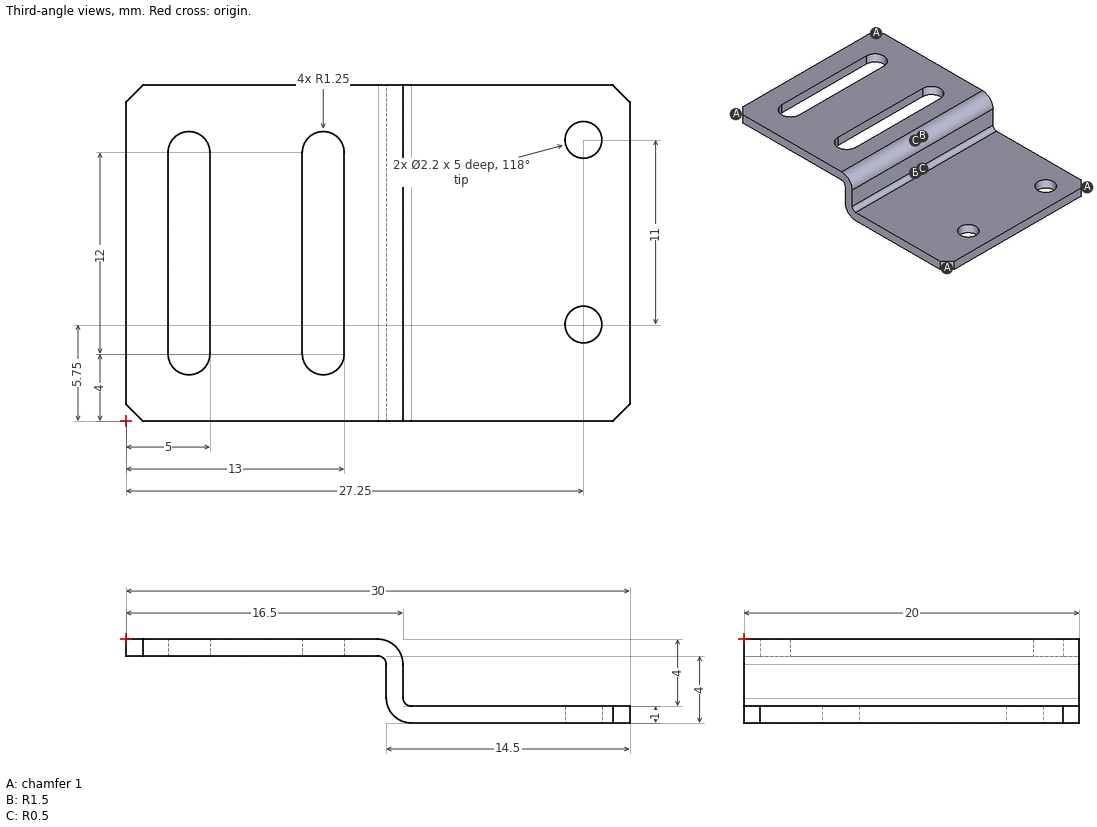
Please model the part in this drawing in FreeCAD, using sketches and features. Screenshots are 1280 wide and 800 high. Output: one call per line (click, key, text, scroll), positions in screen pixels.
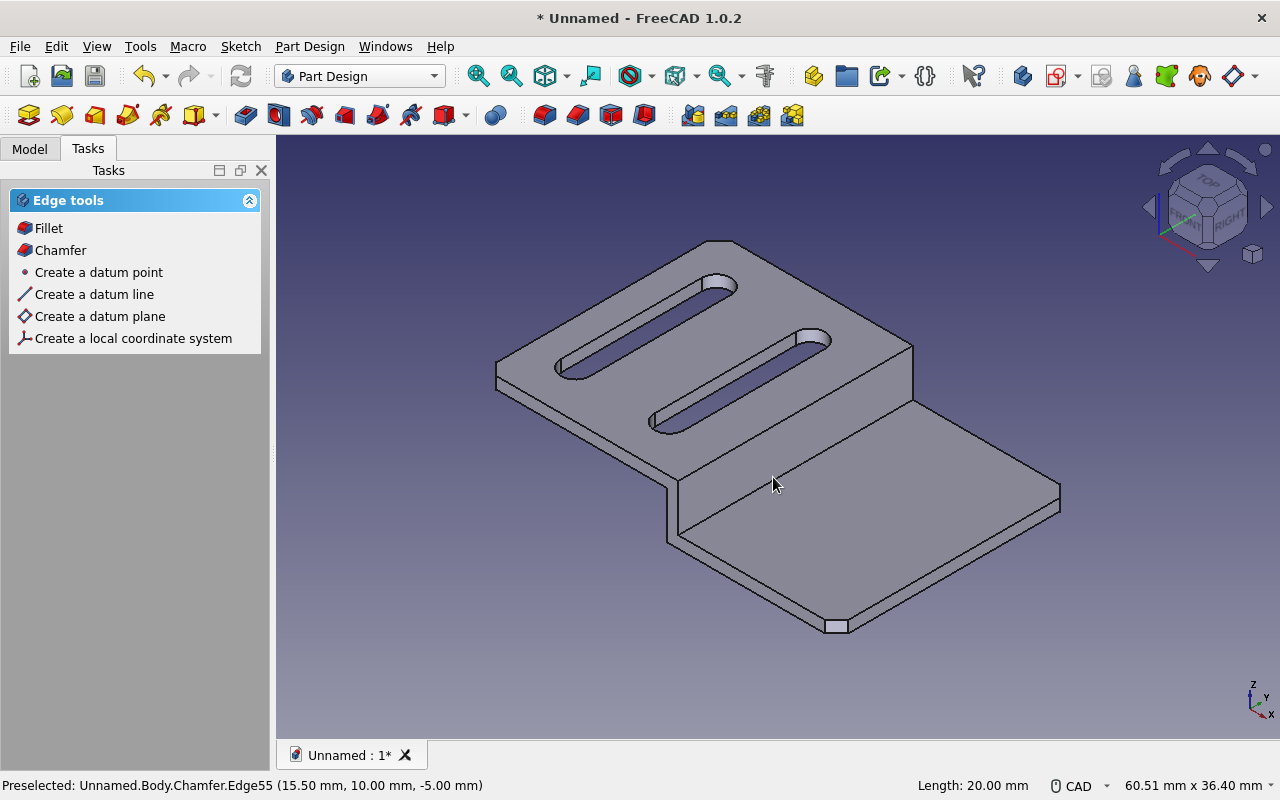
click(796, 412, ctrl)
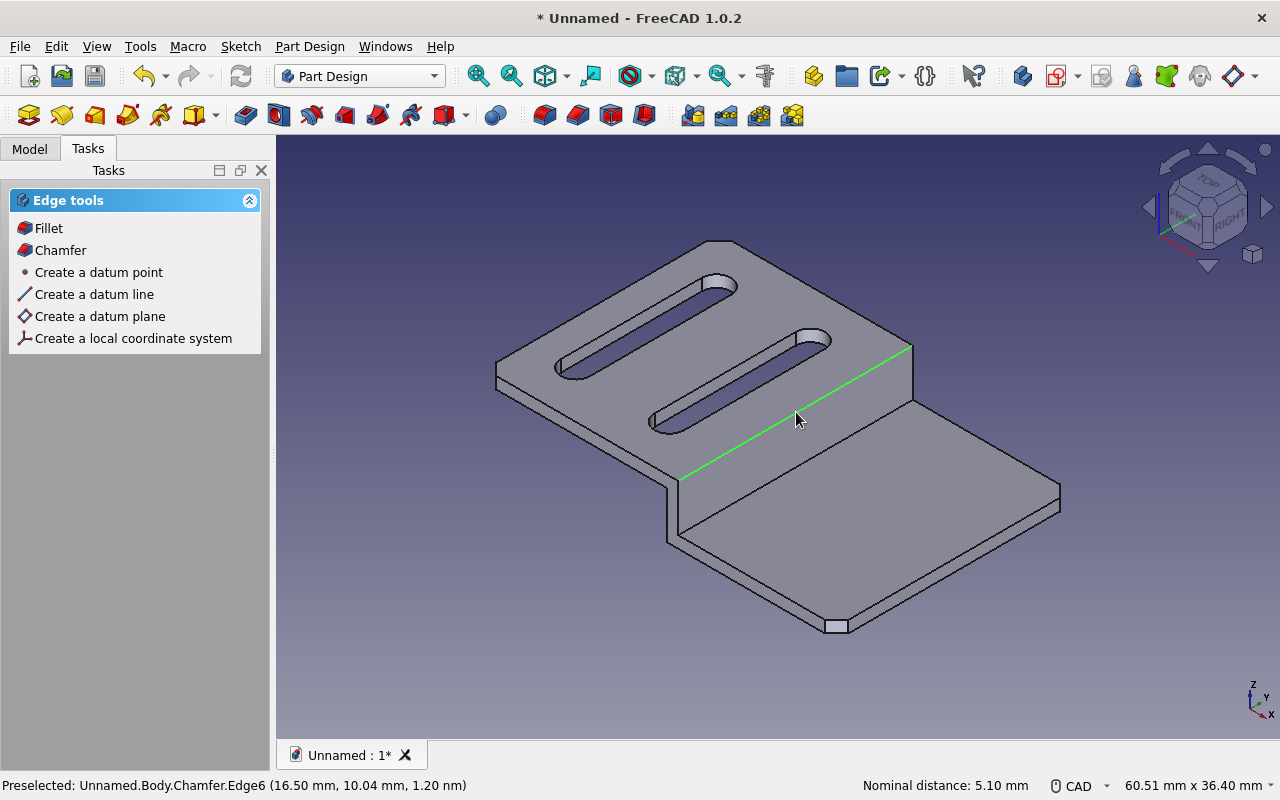
click(545, 116)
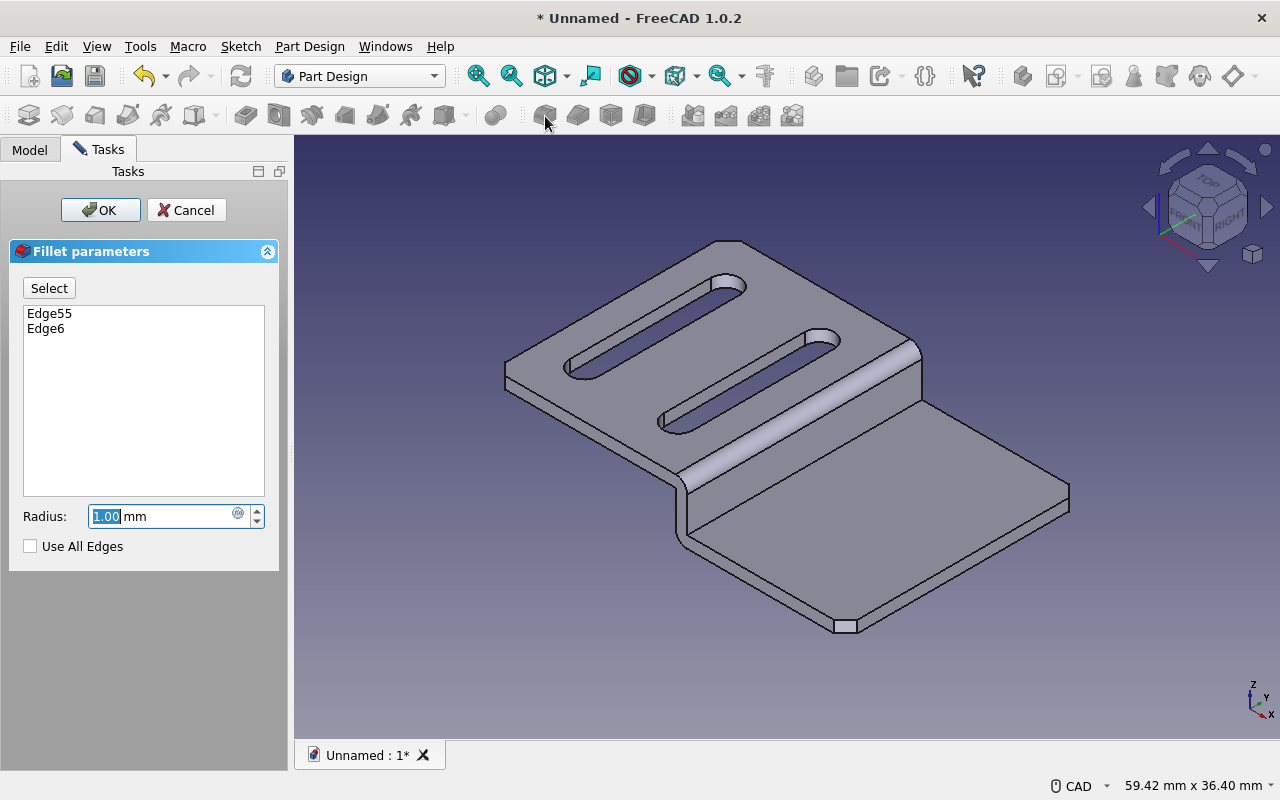
text(1.5)
key(Tab)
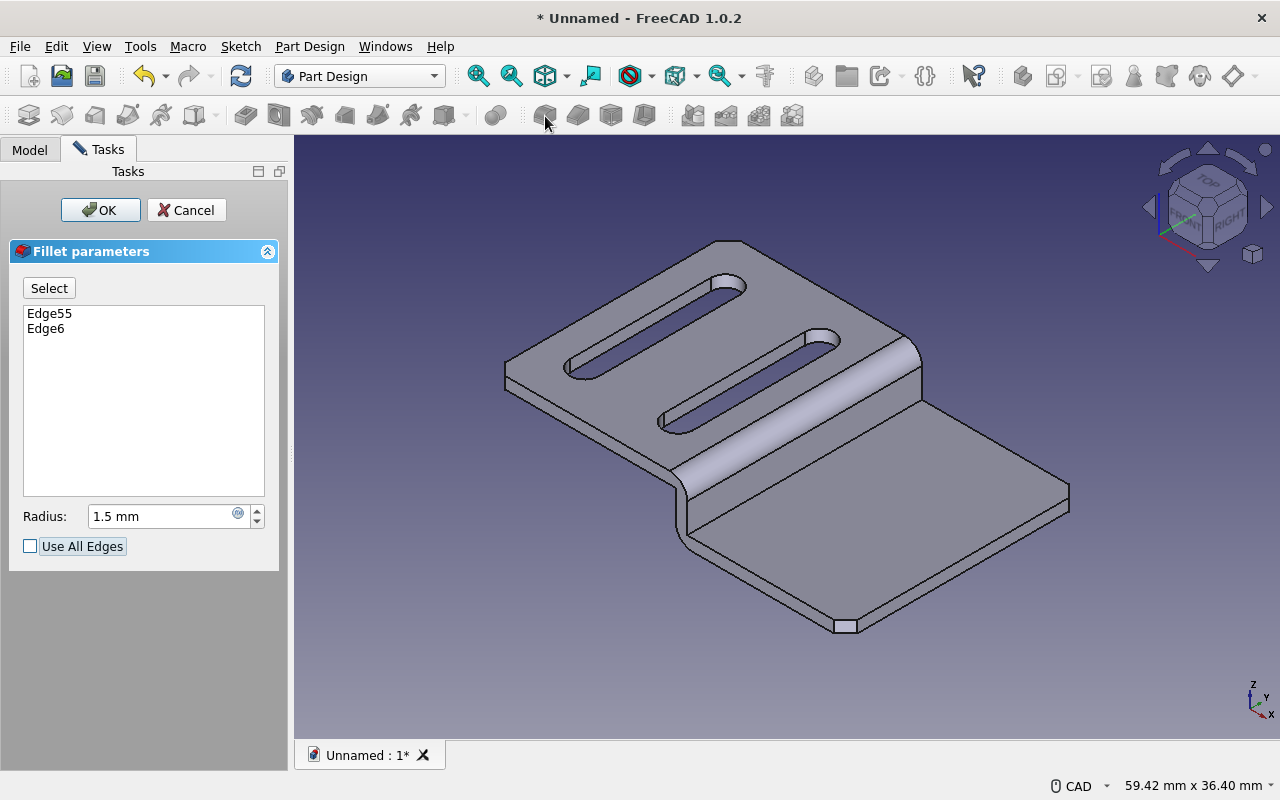
click(101, 210)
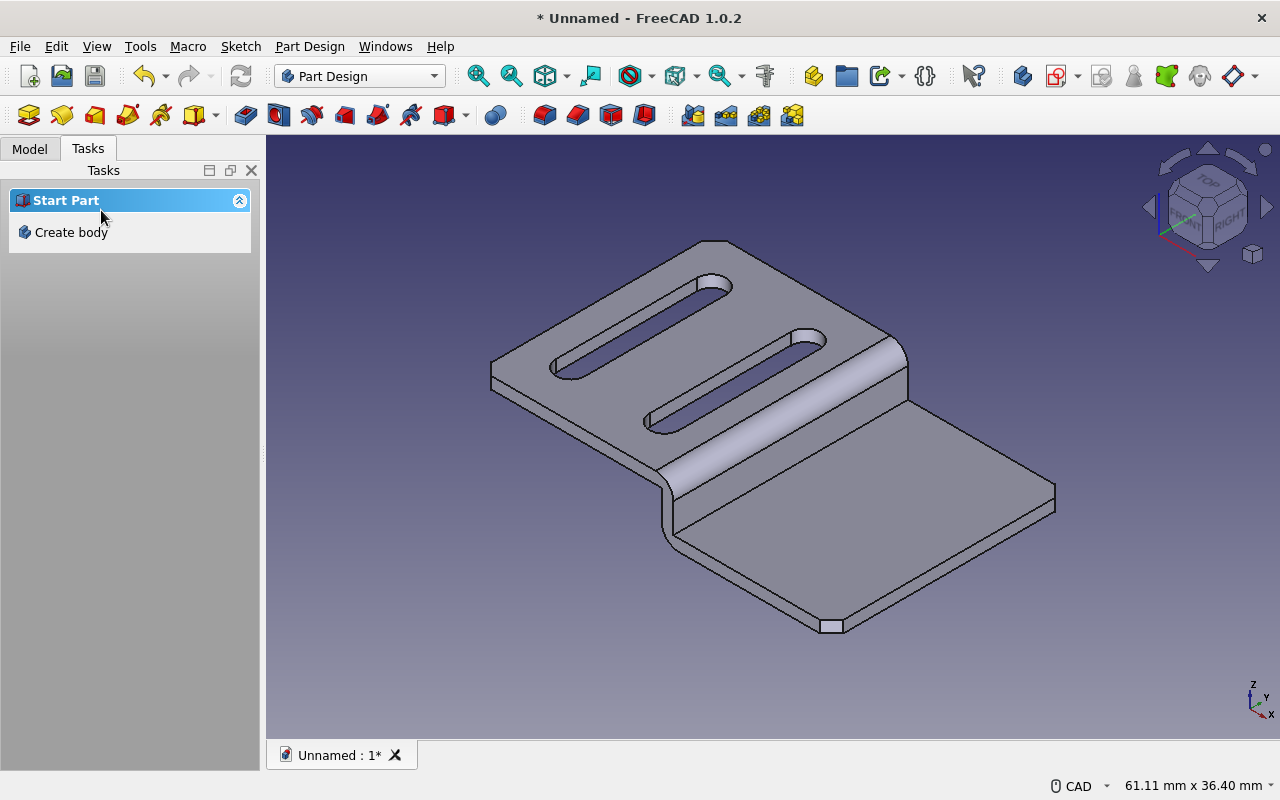
key(2)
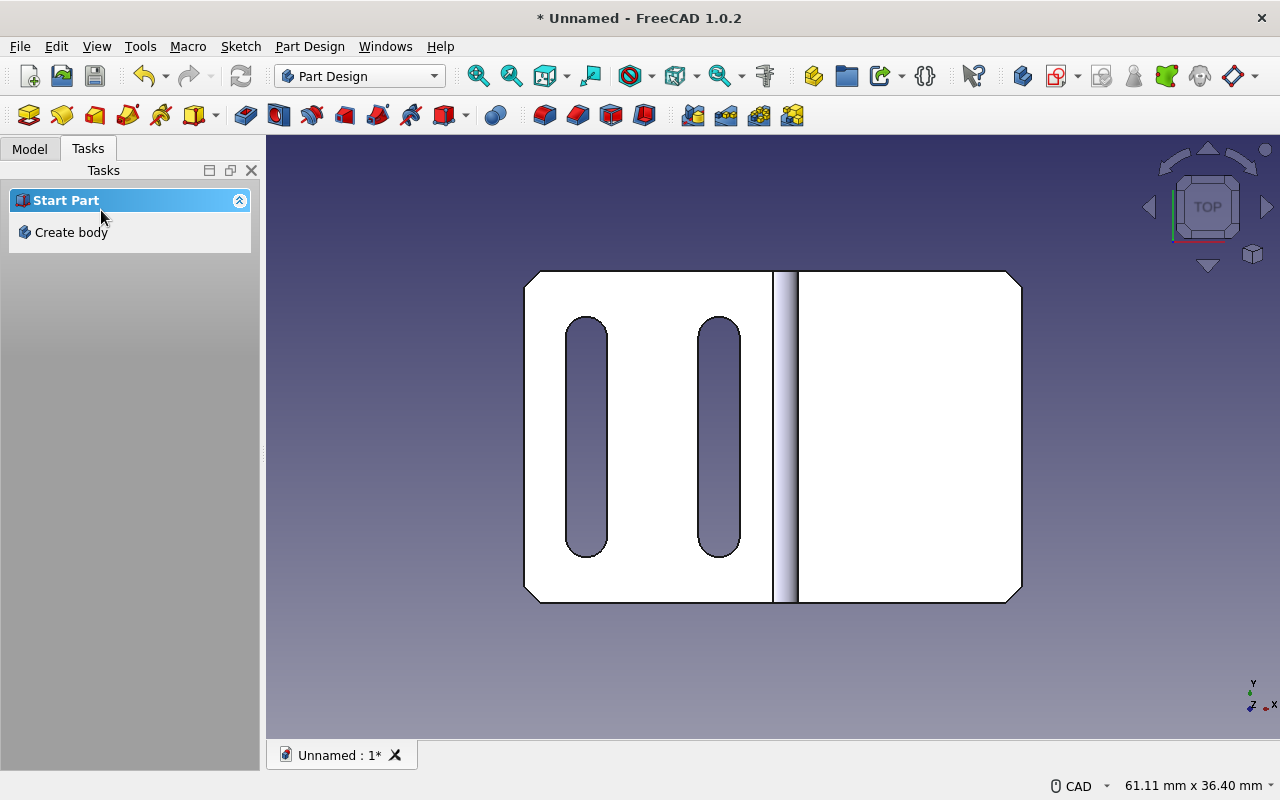
key(0)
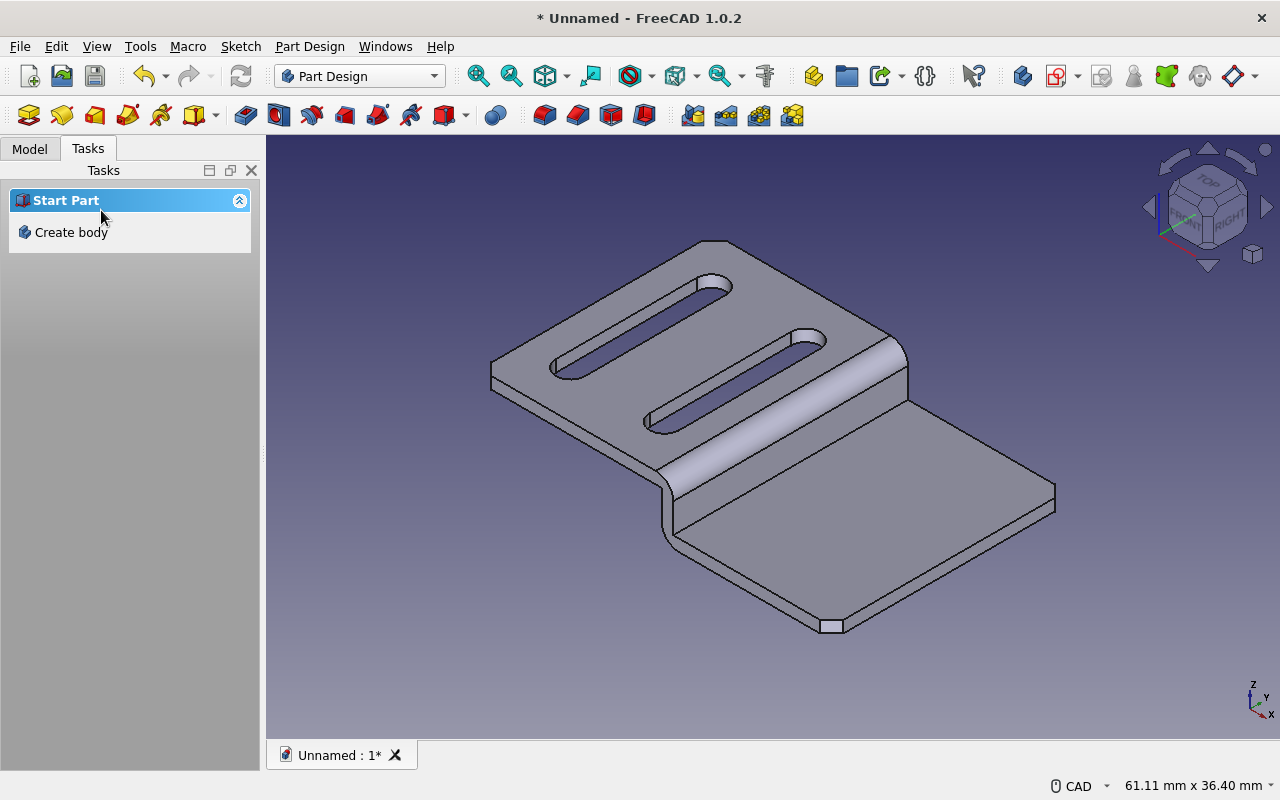
key(1)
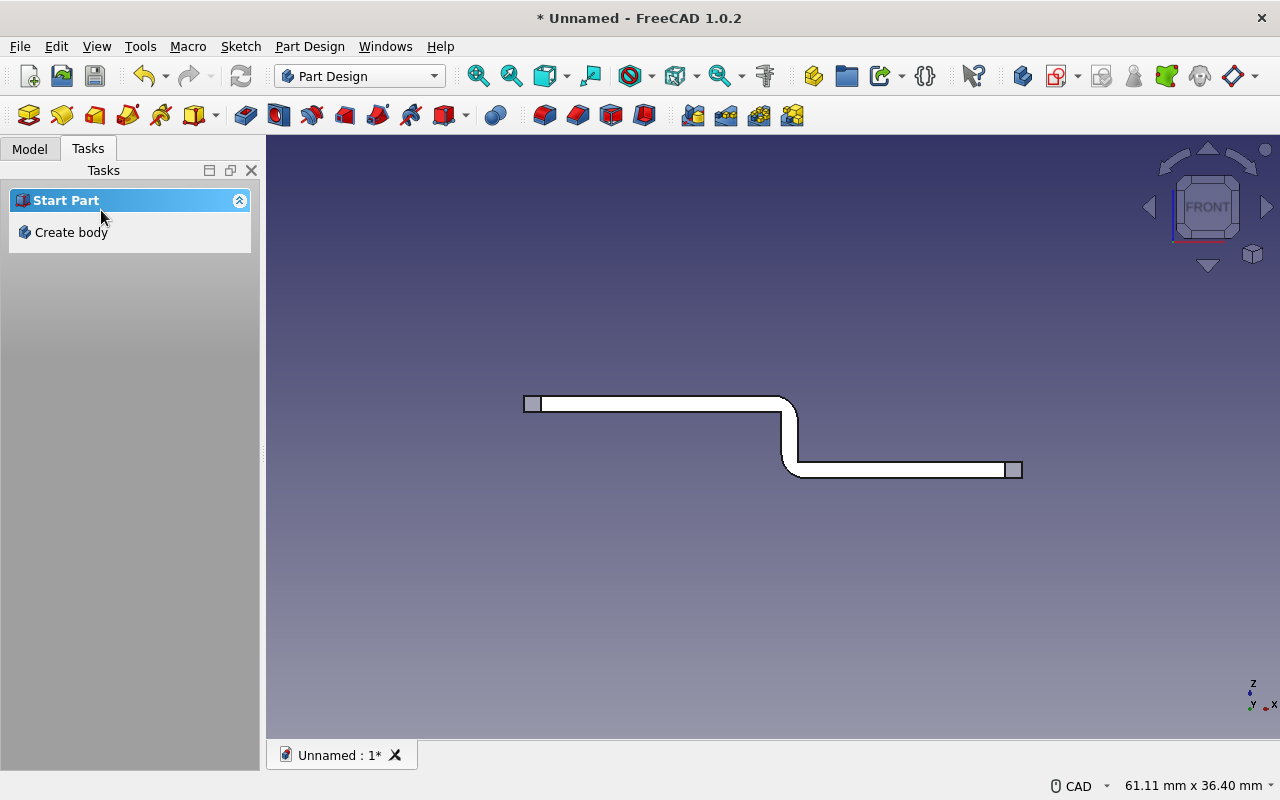
key(3)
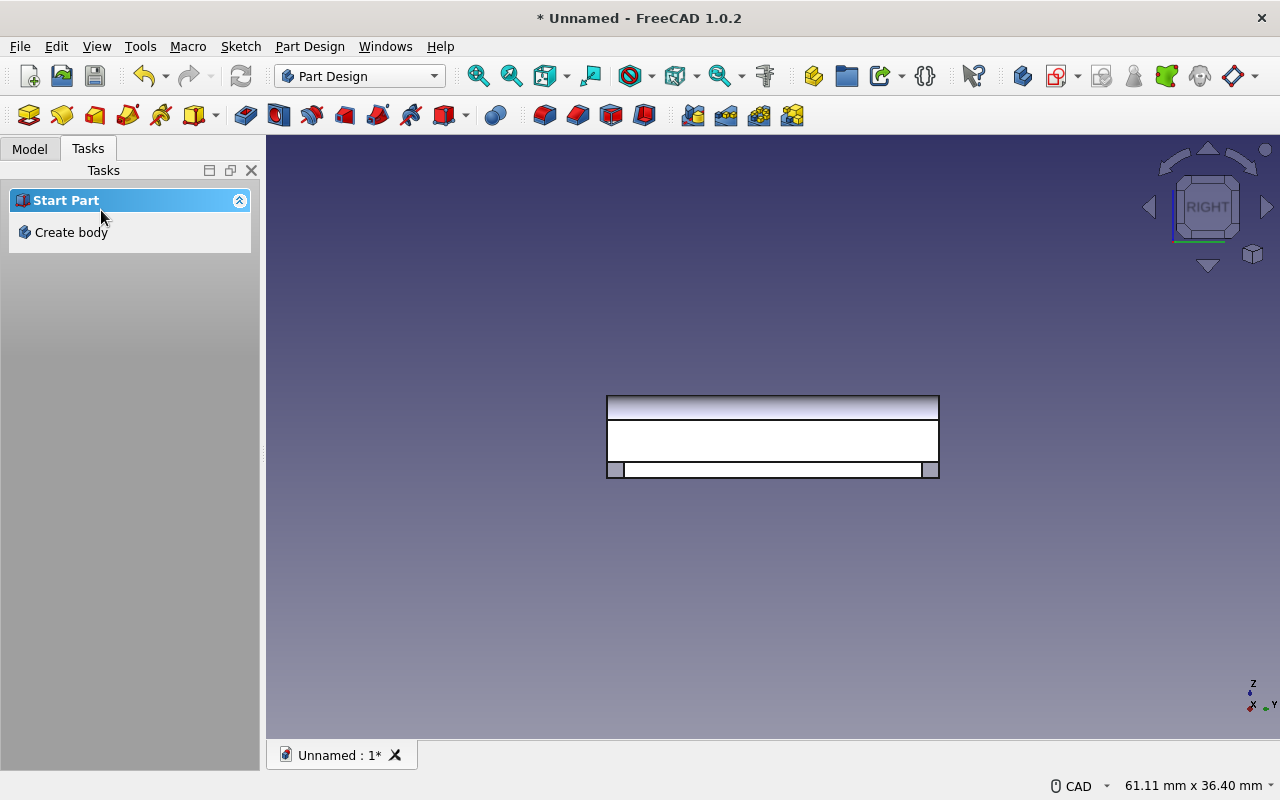
click(479, 76)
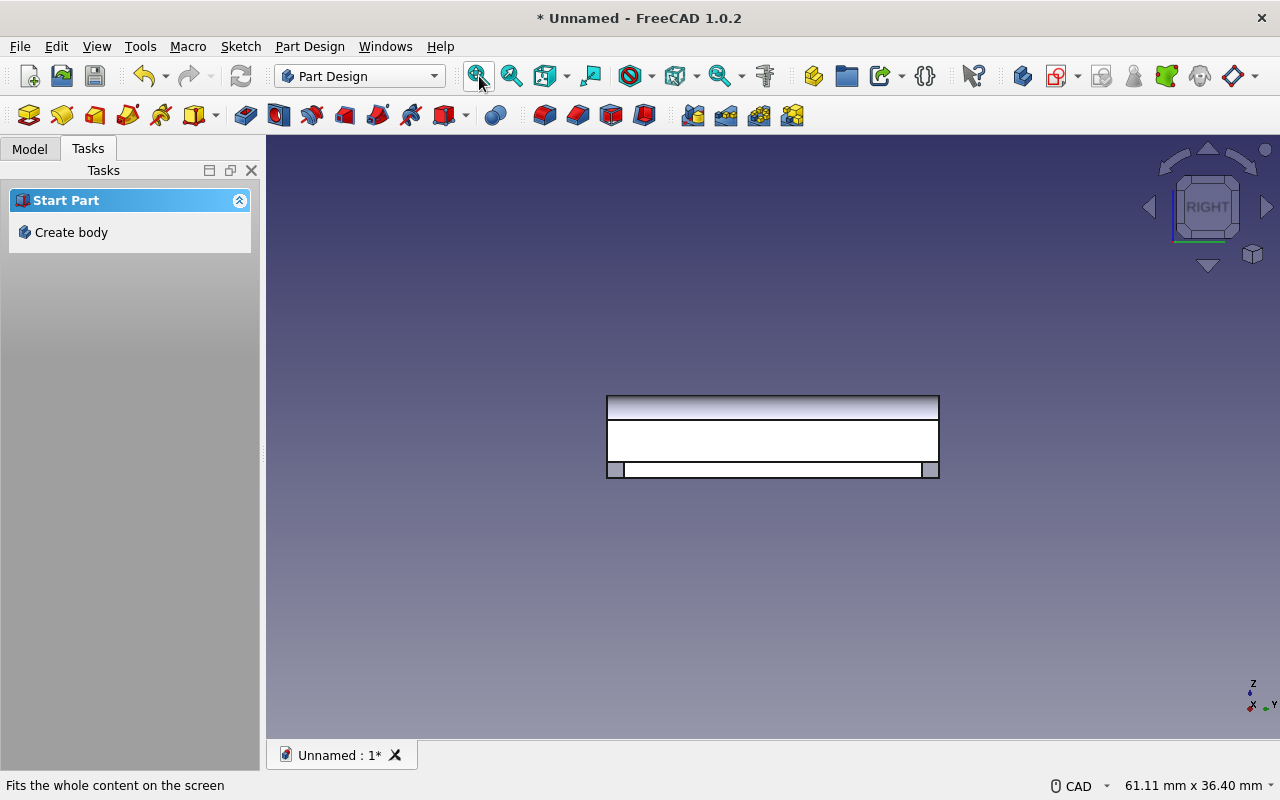
key(5)